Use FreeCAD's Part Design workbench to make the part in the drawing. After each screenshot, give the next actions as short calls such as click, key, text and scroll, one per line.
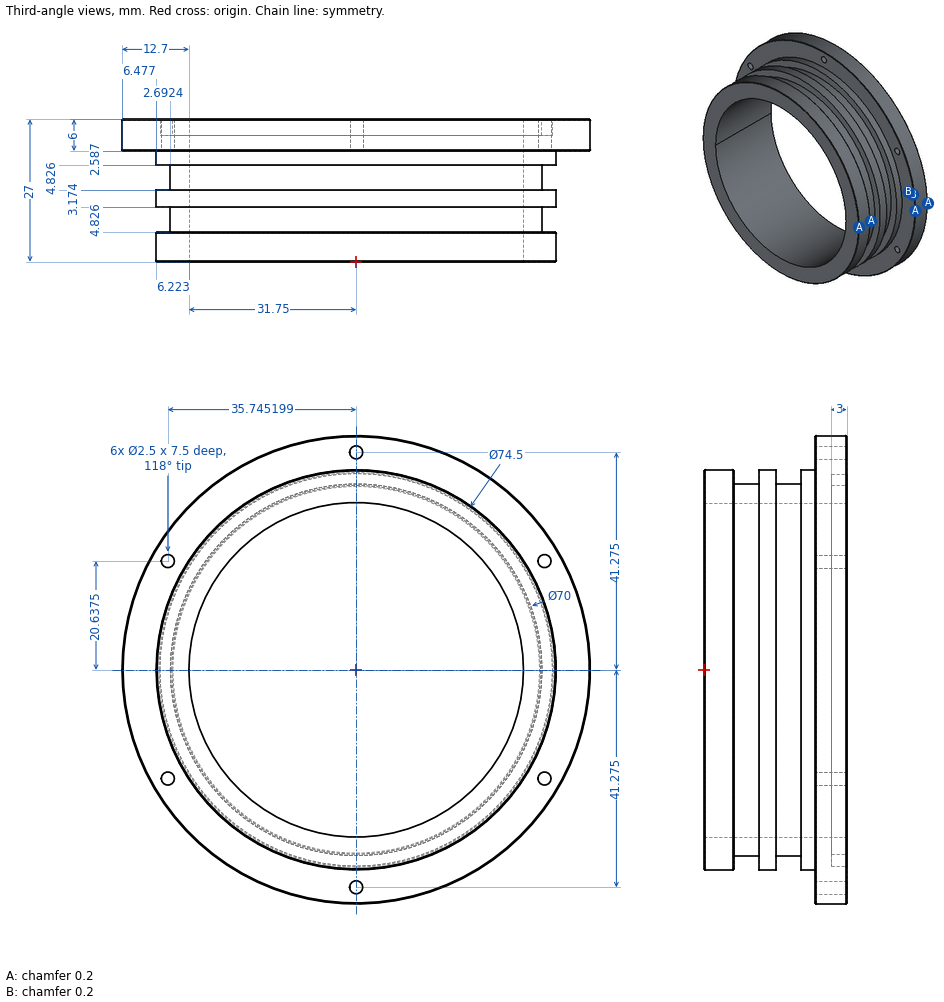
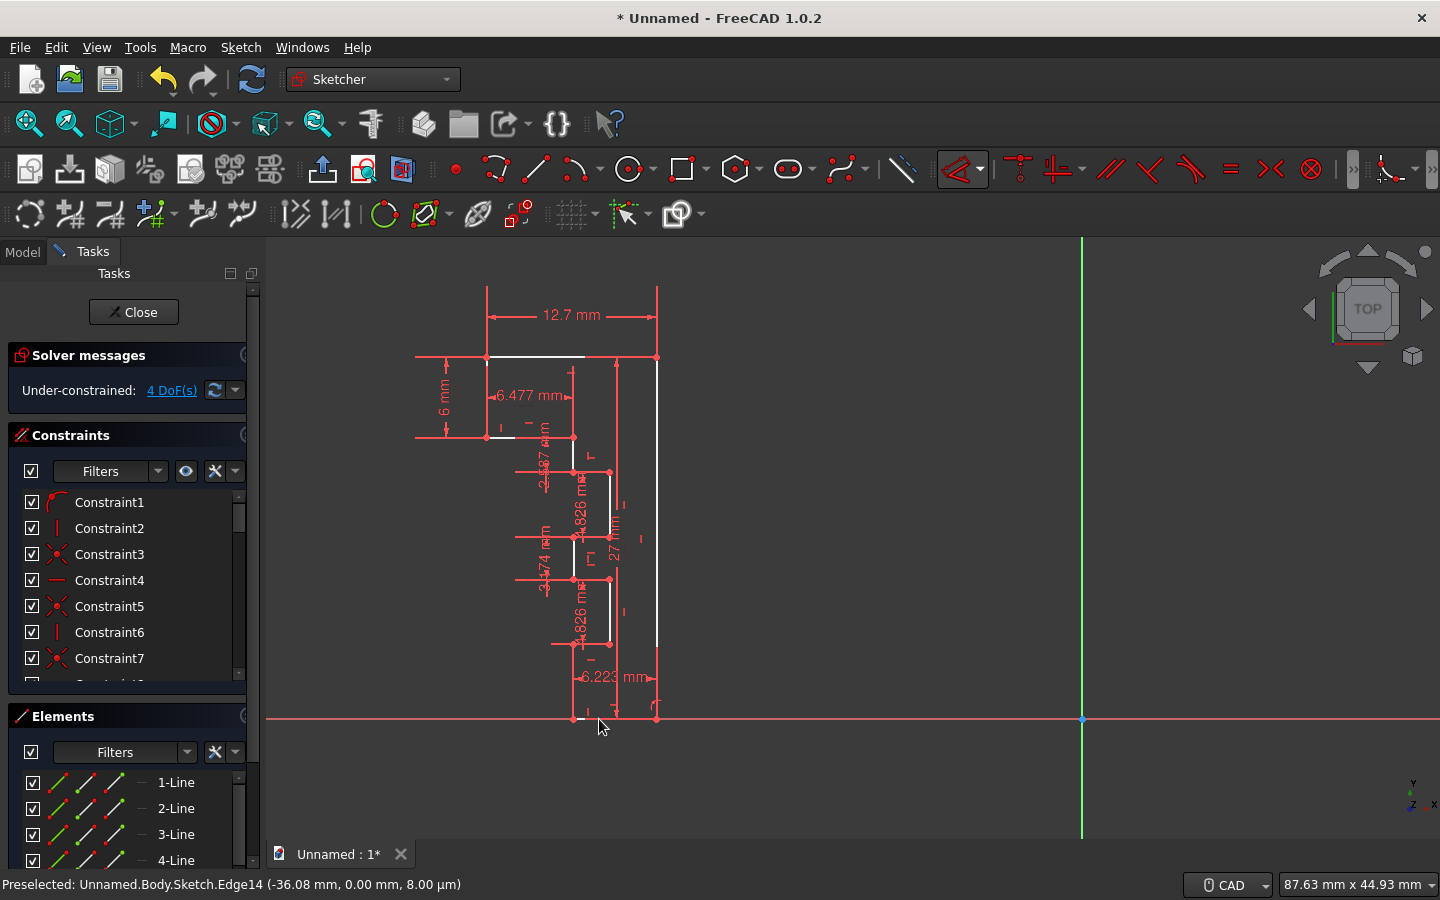
scroll(584, 472, up, 2)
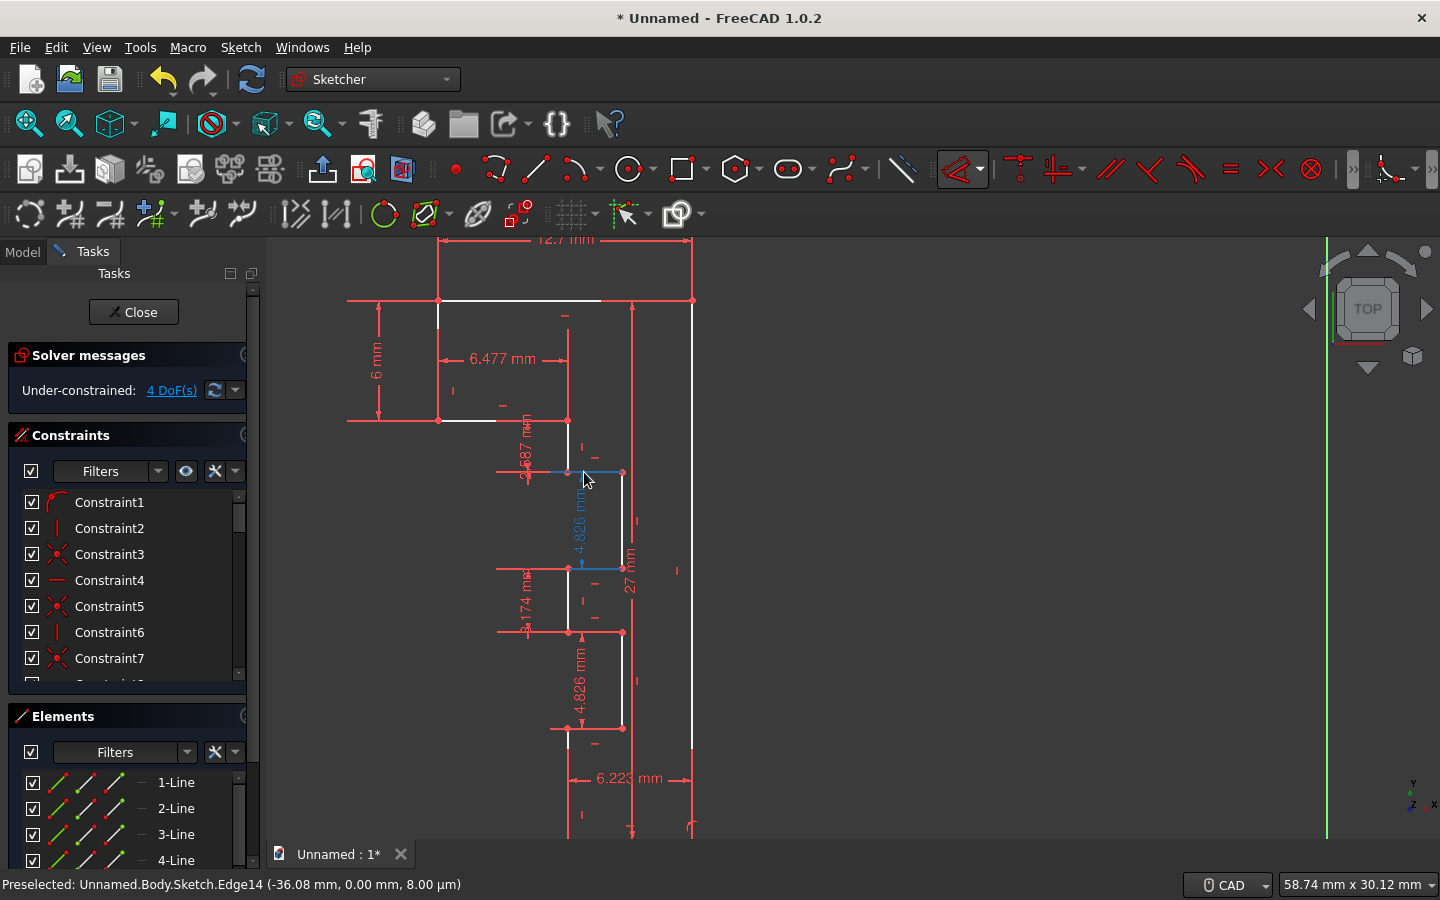
click(584, 472)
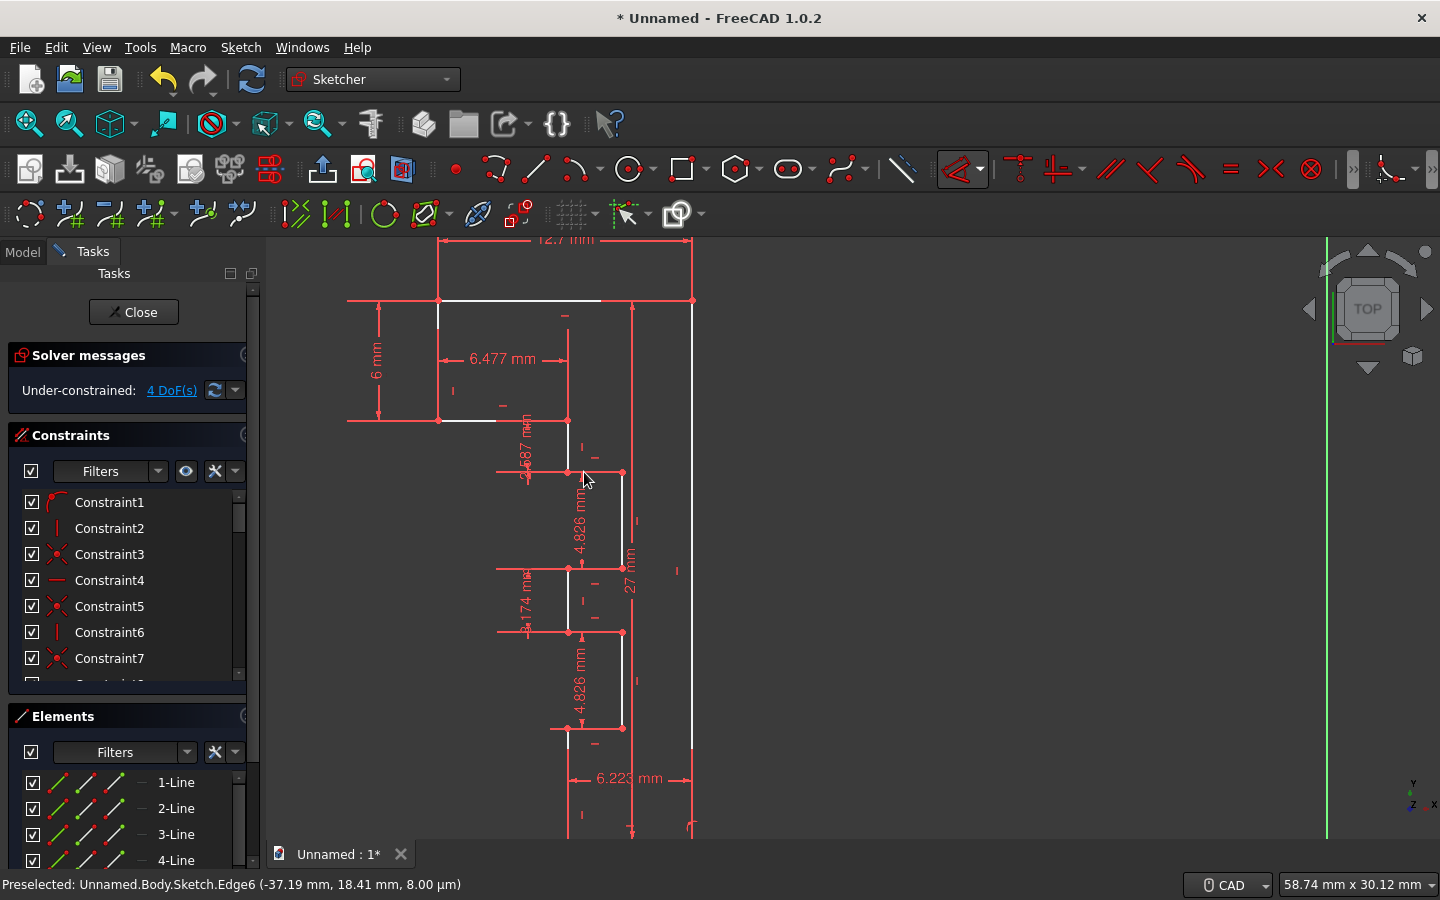
key(l)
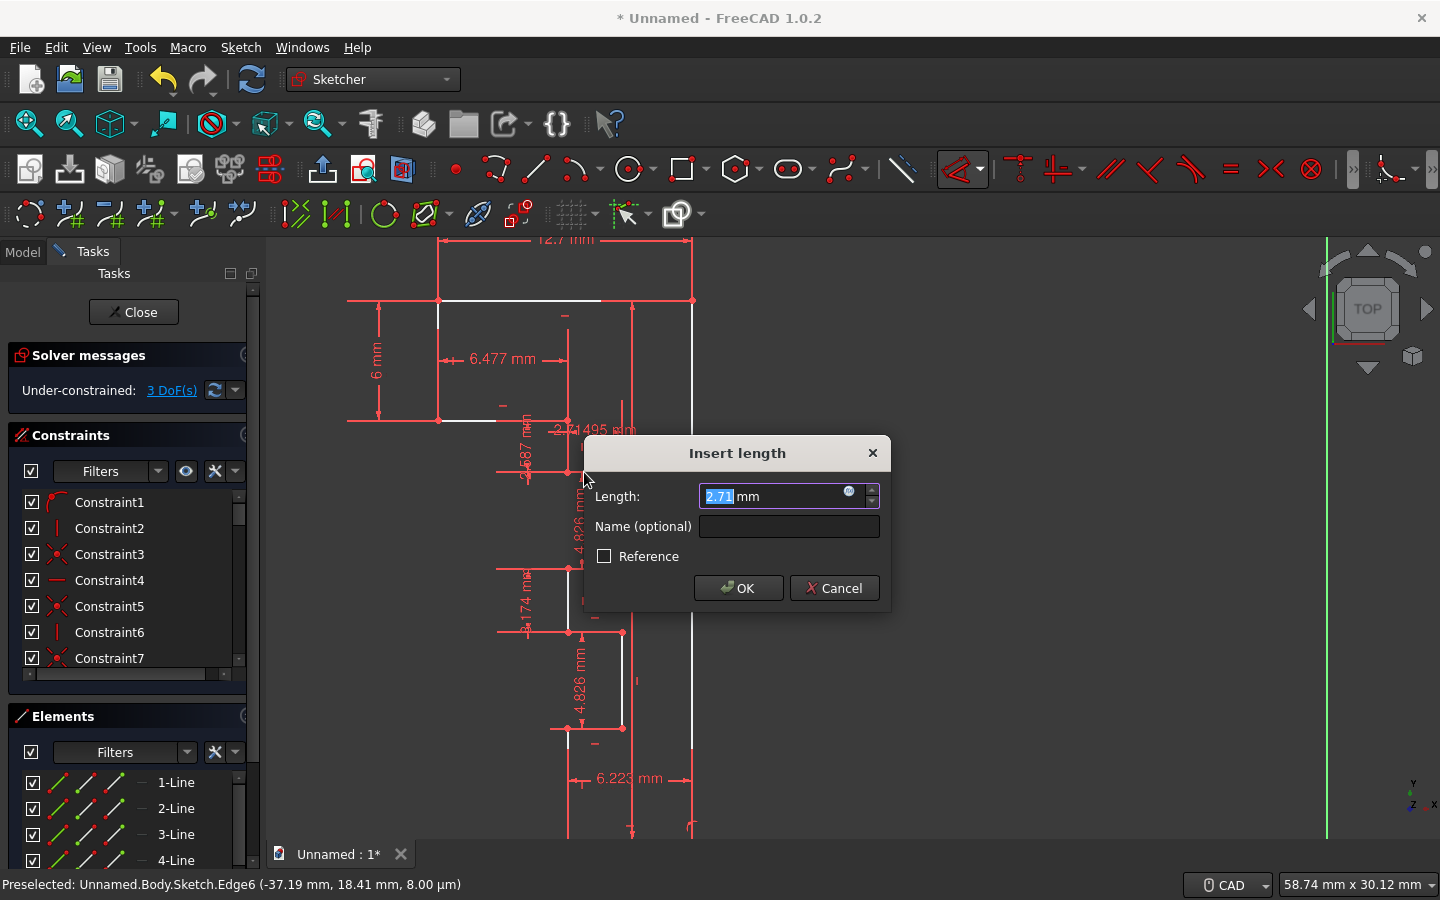
text(2.6924)
key(Return)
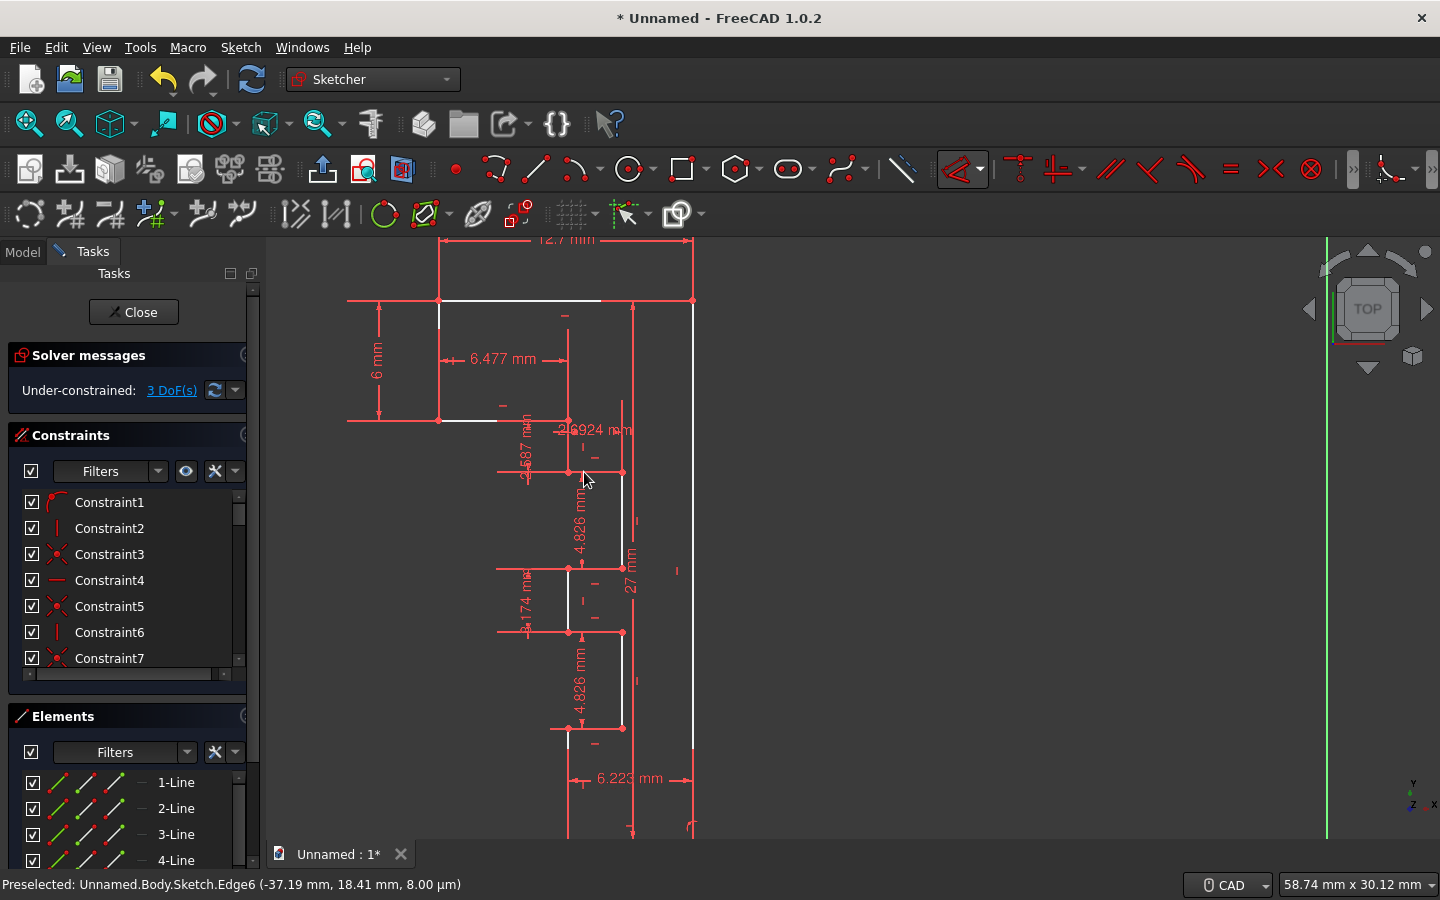
click(606, 569)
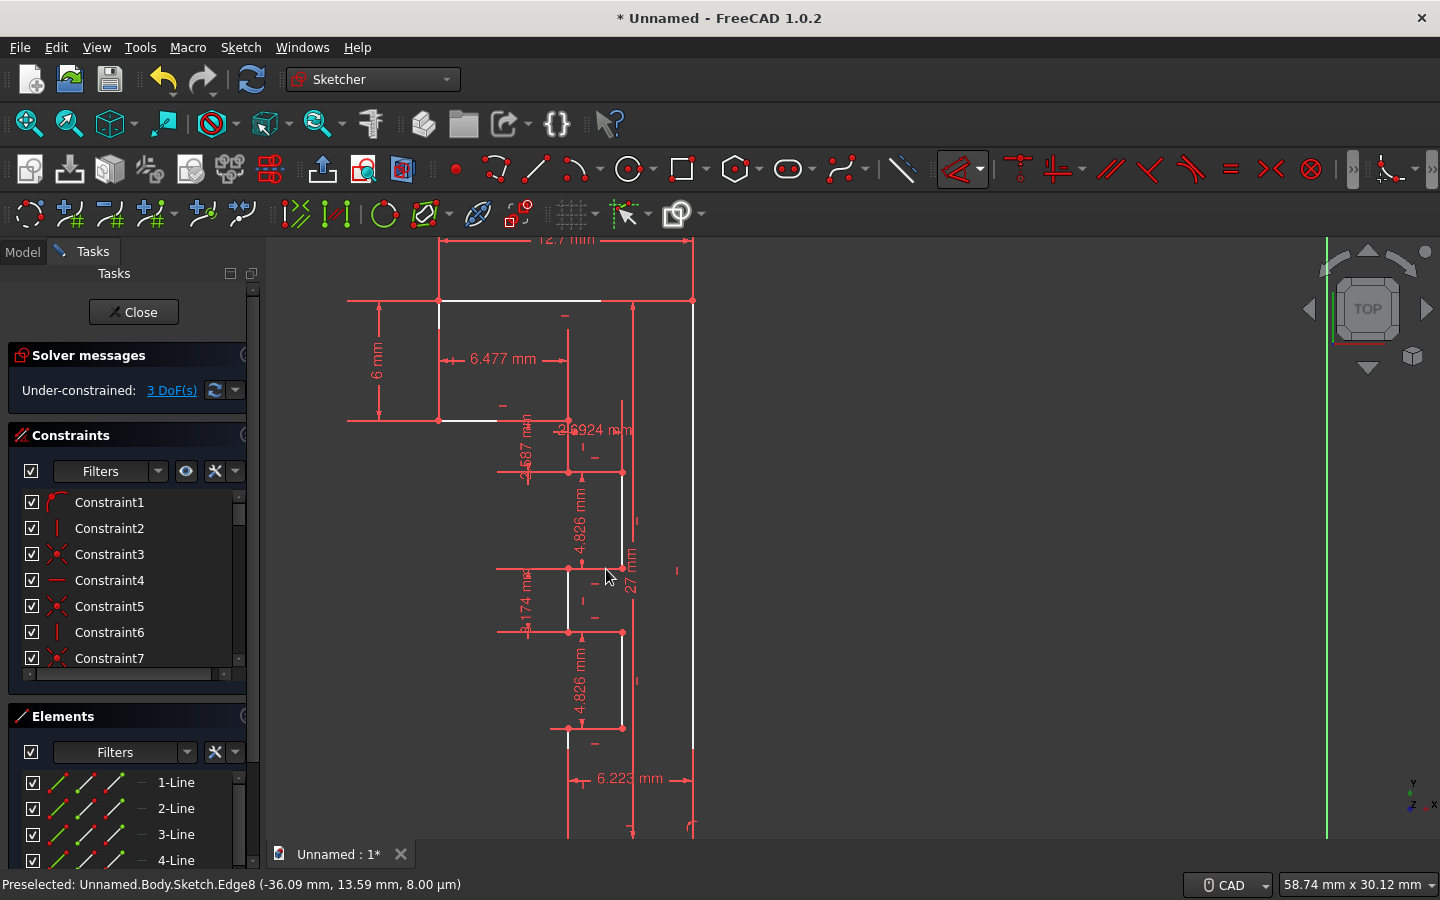
key(l)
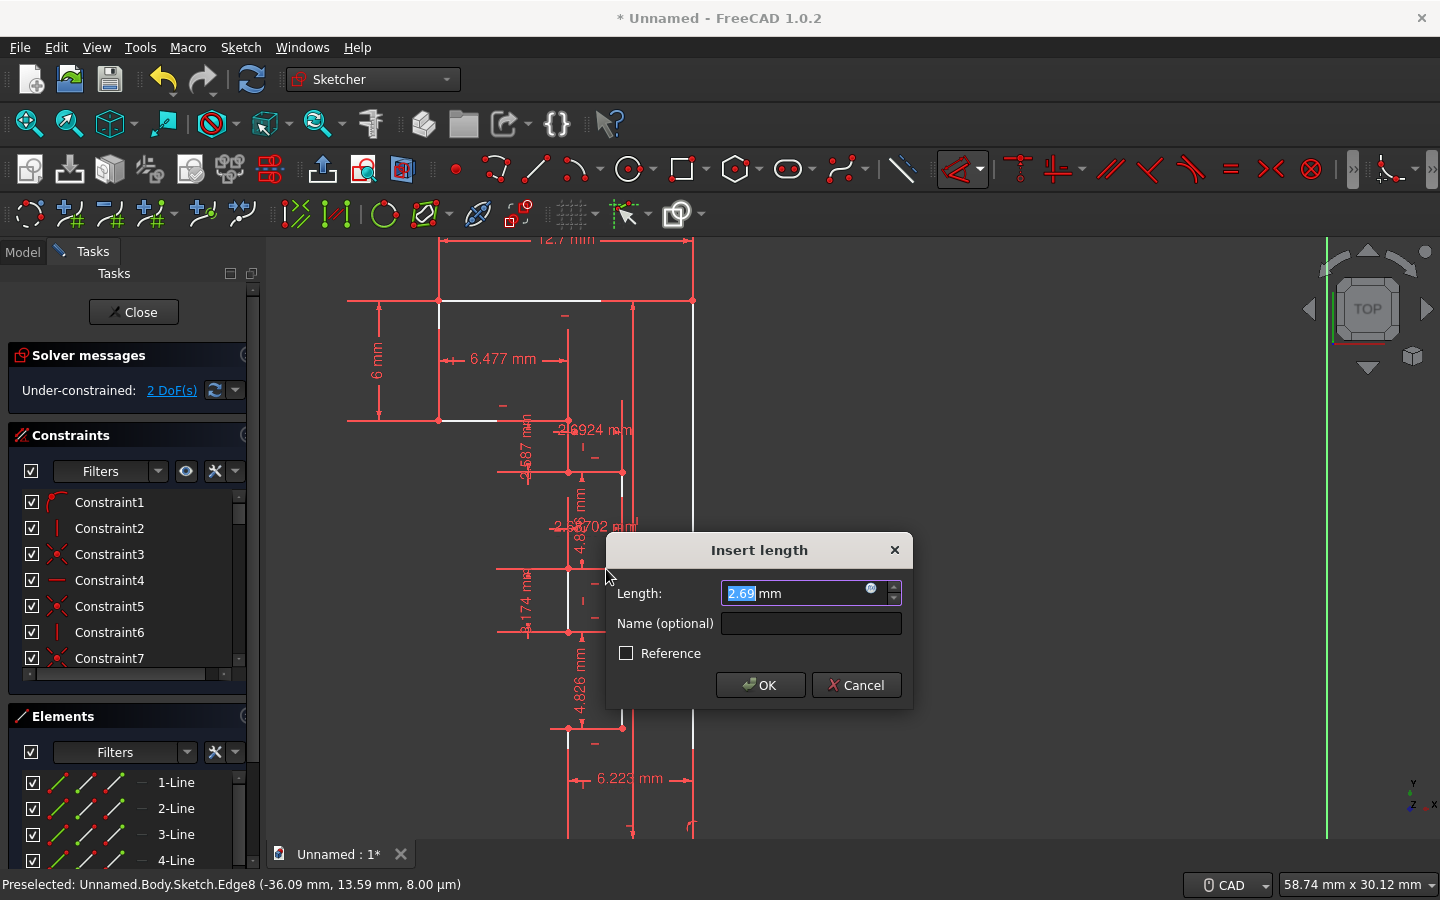
text(2.6924)
key(Return)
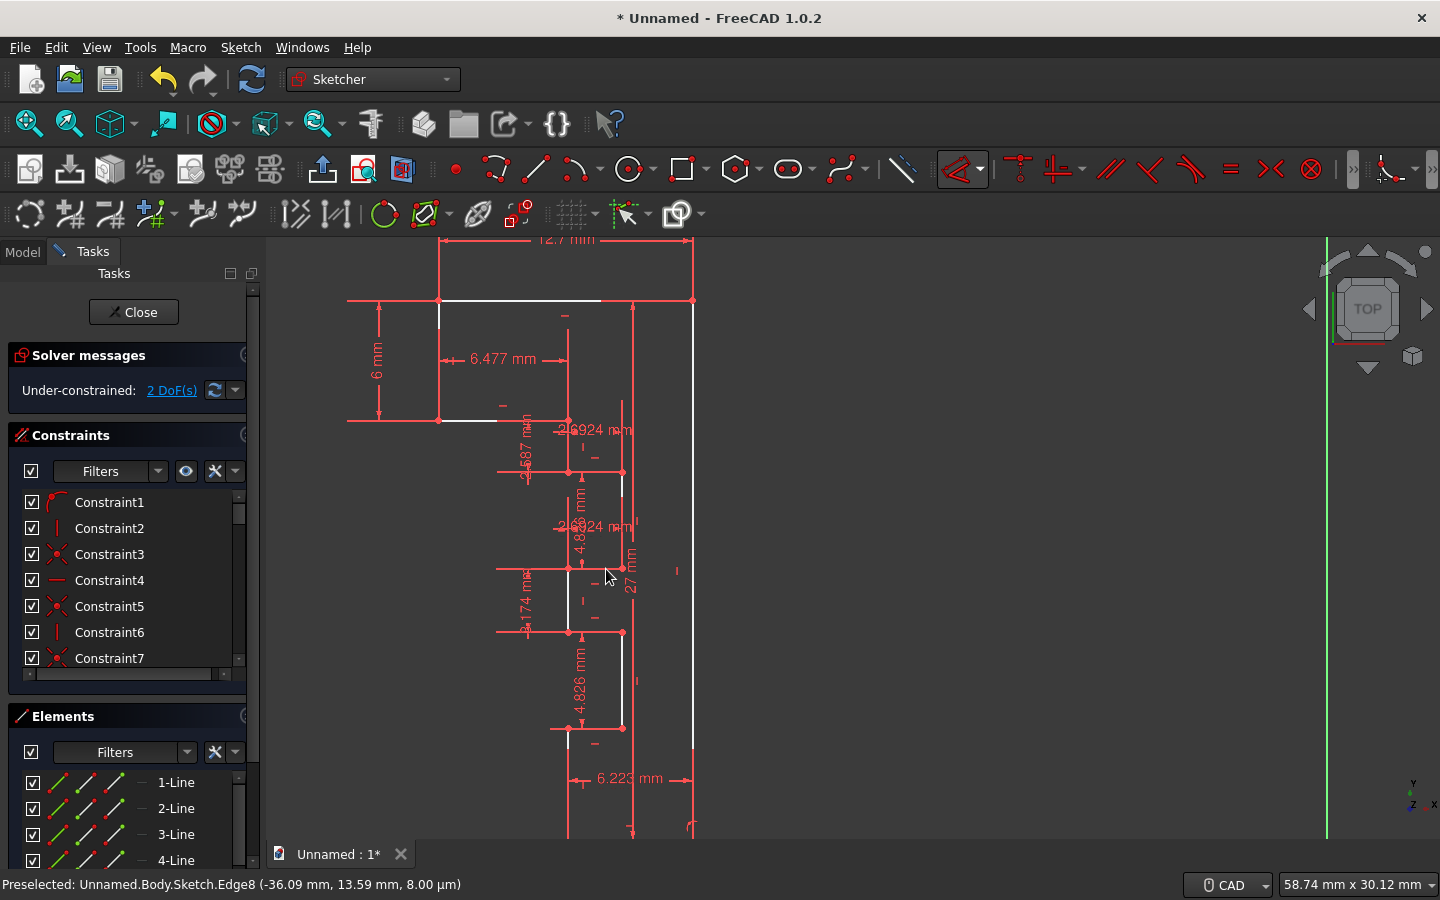
click(584, 632)